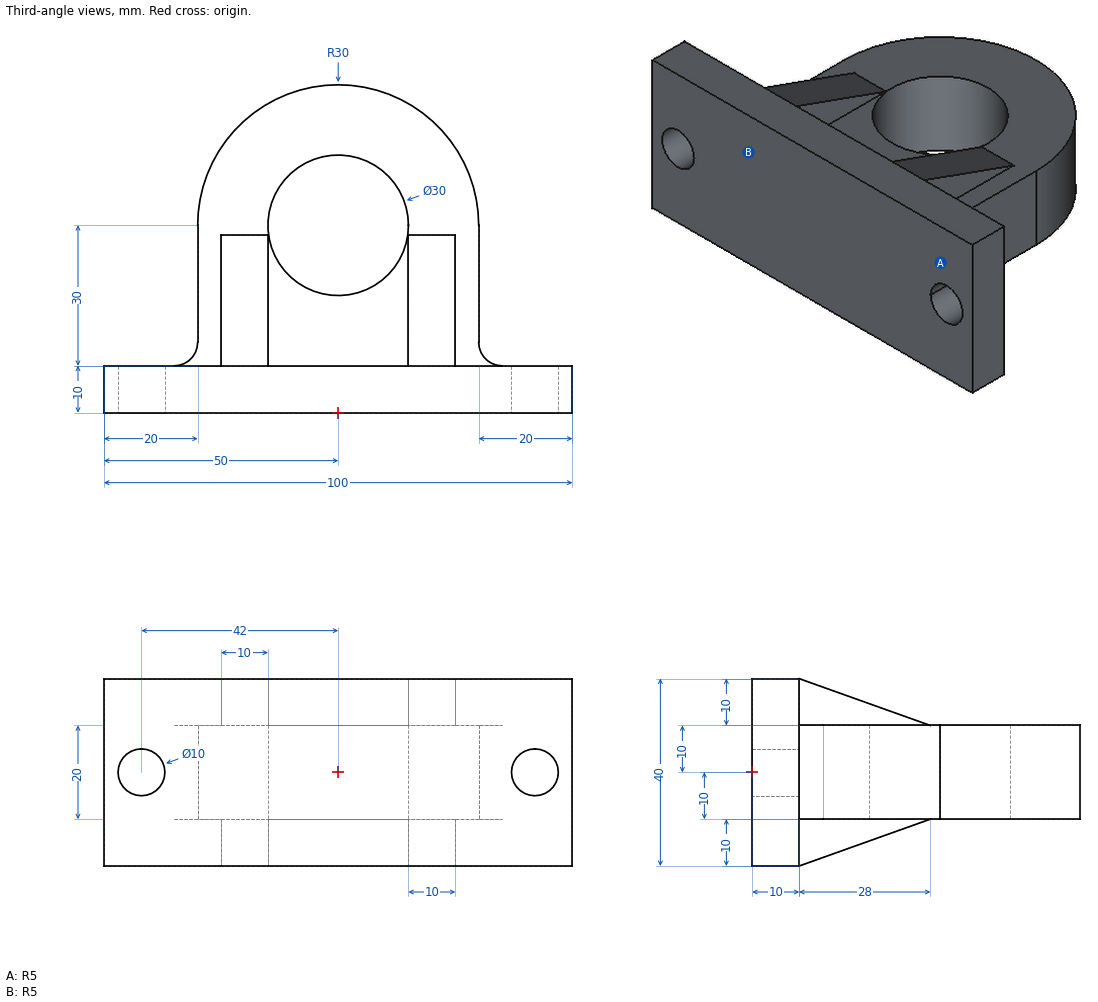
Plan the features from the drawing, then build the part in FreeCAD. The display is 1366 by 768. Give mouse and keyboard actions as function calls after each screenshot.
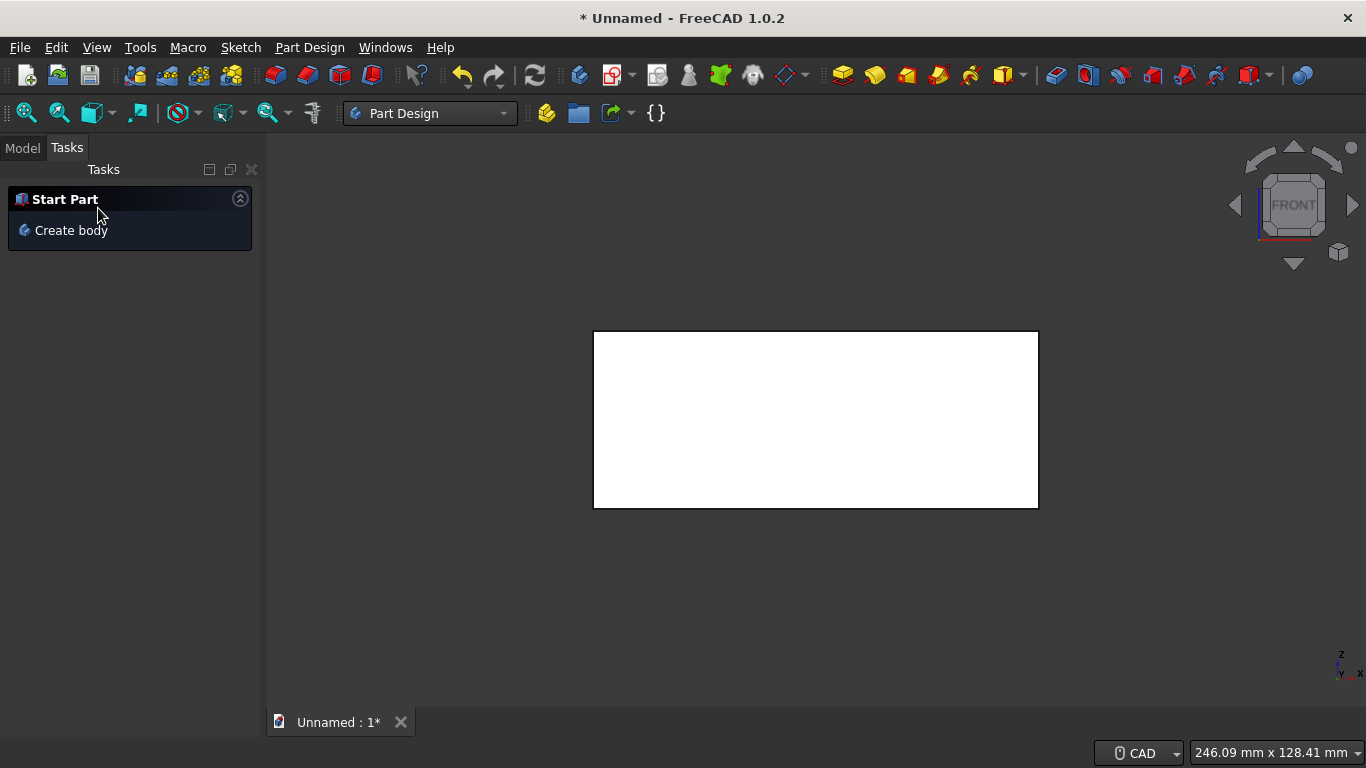
click(28, 114)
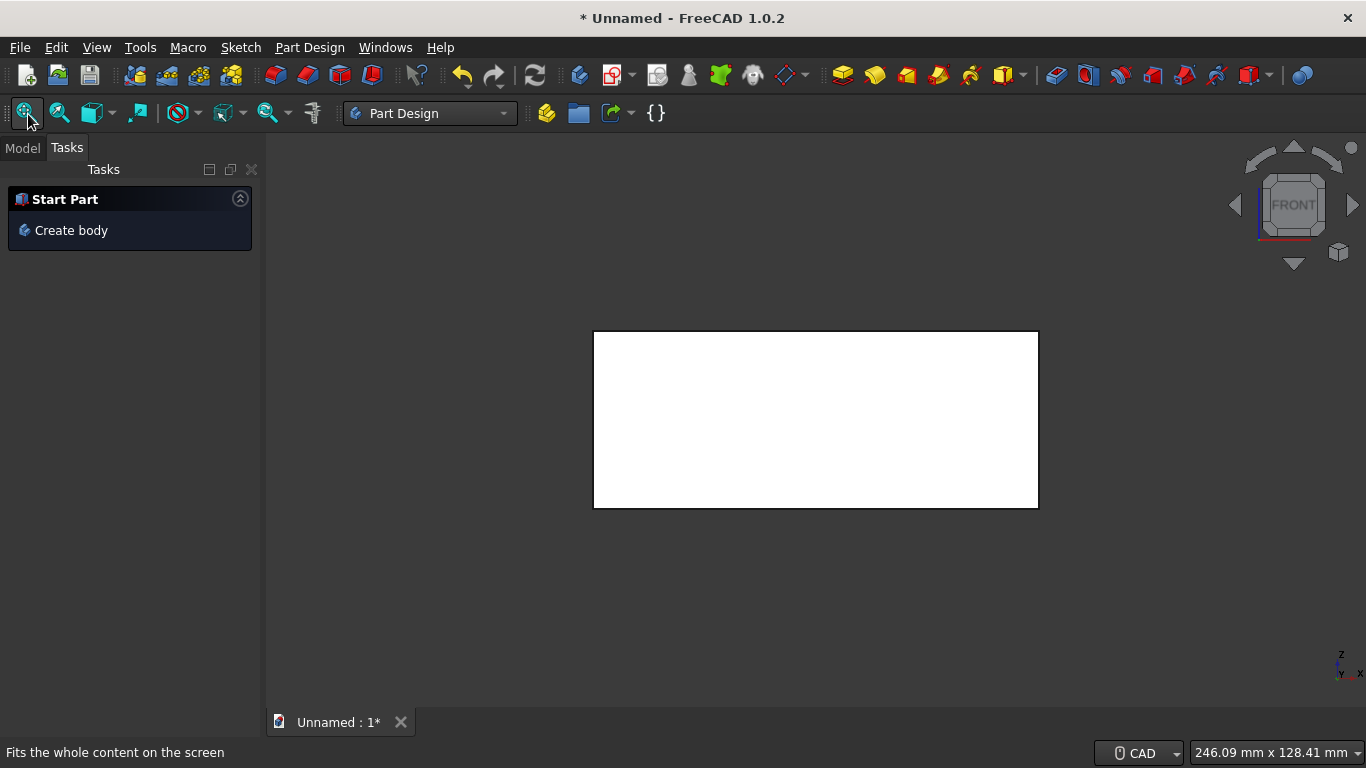
key(3)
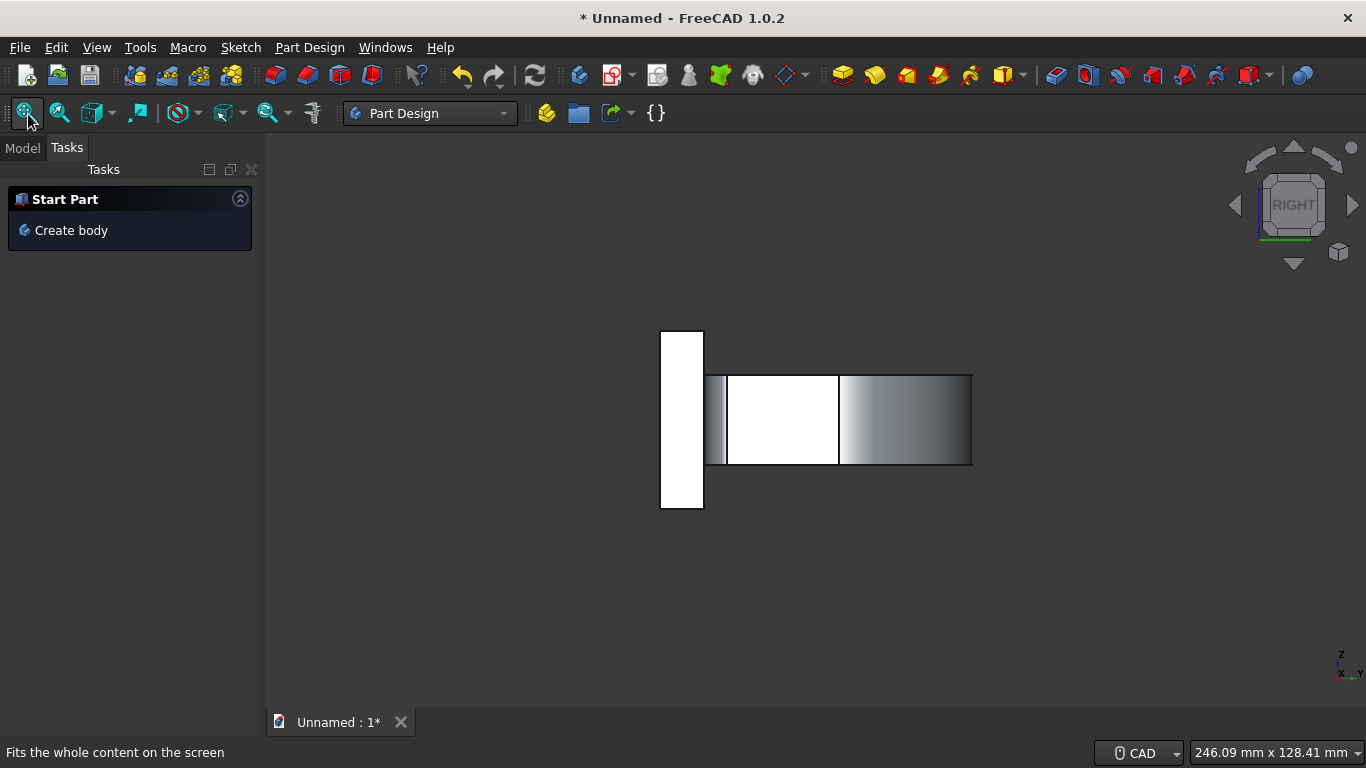
click(28, 114)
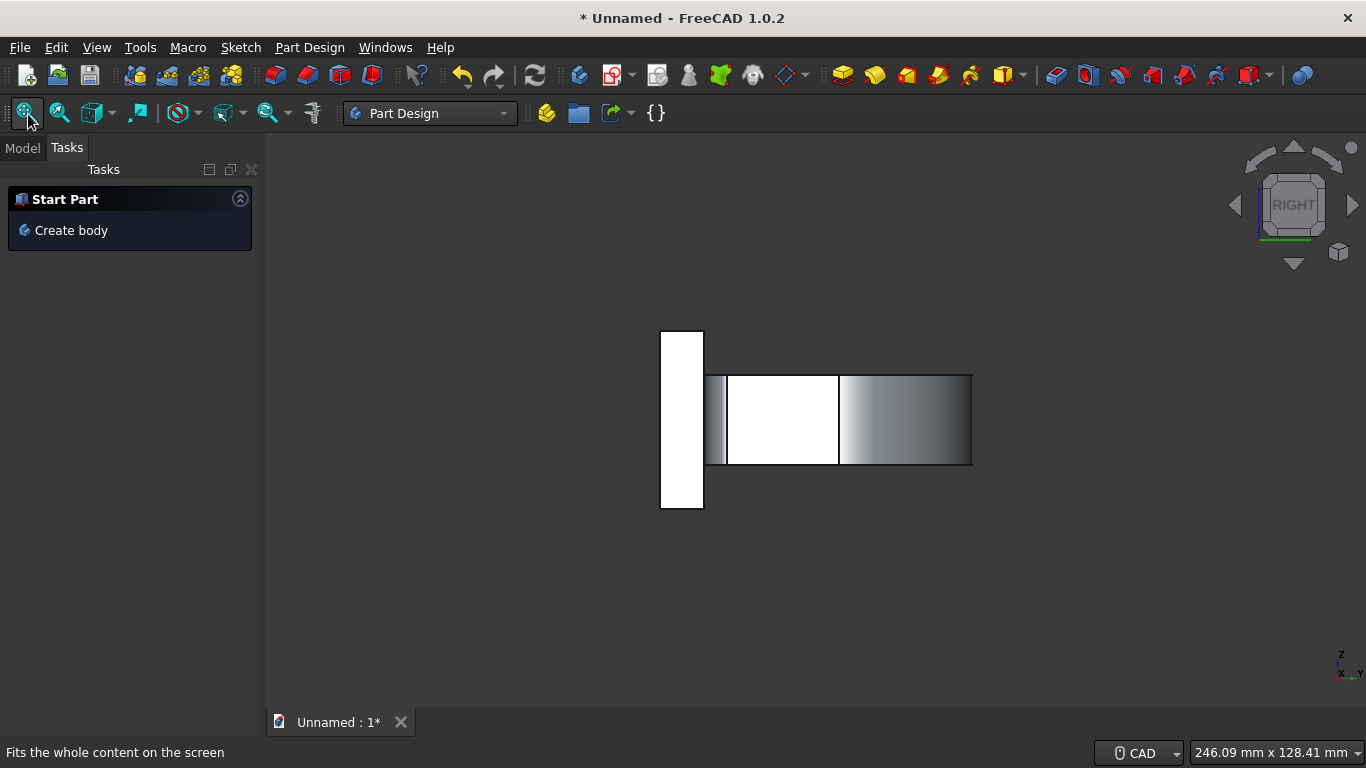
key(5)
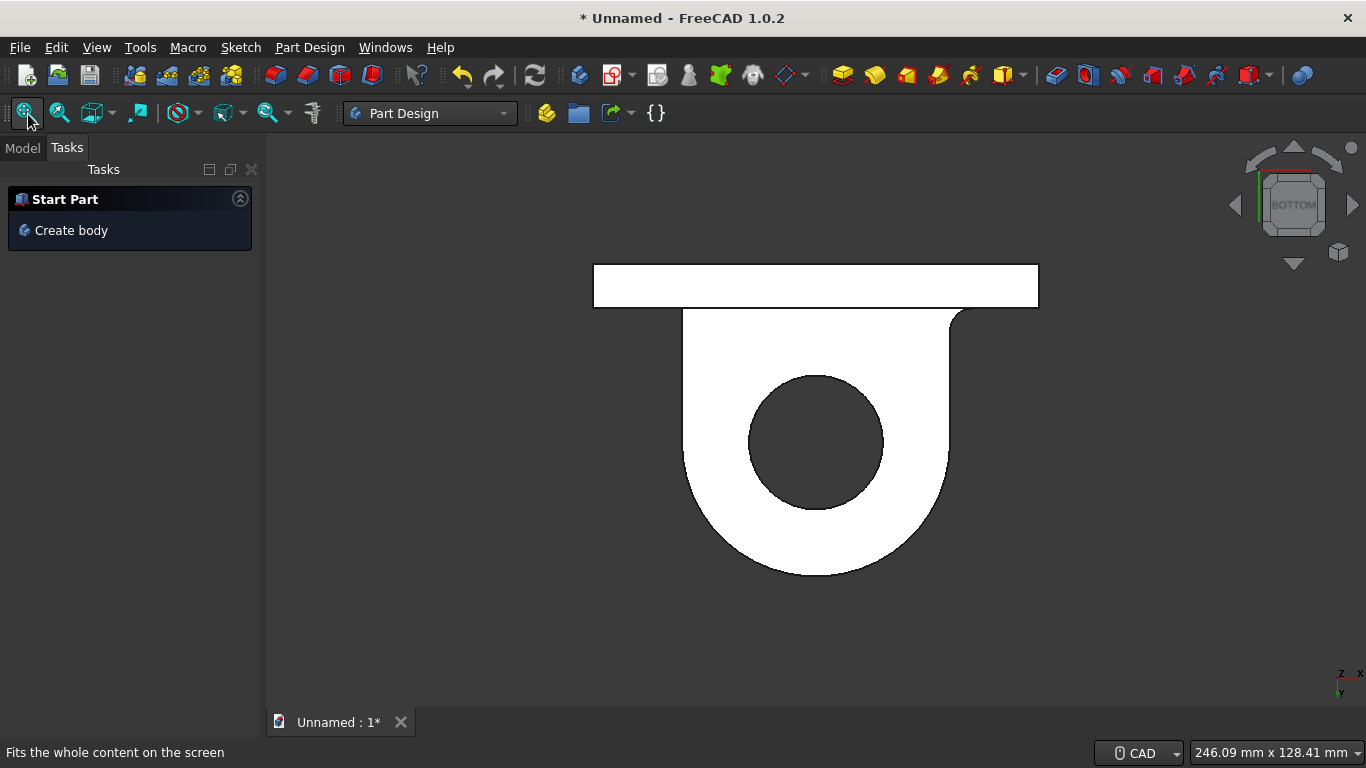
key(4)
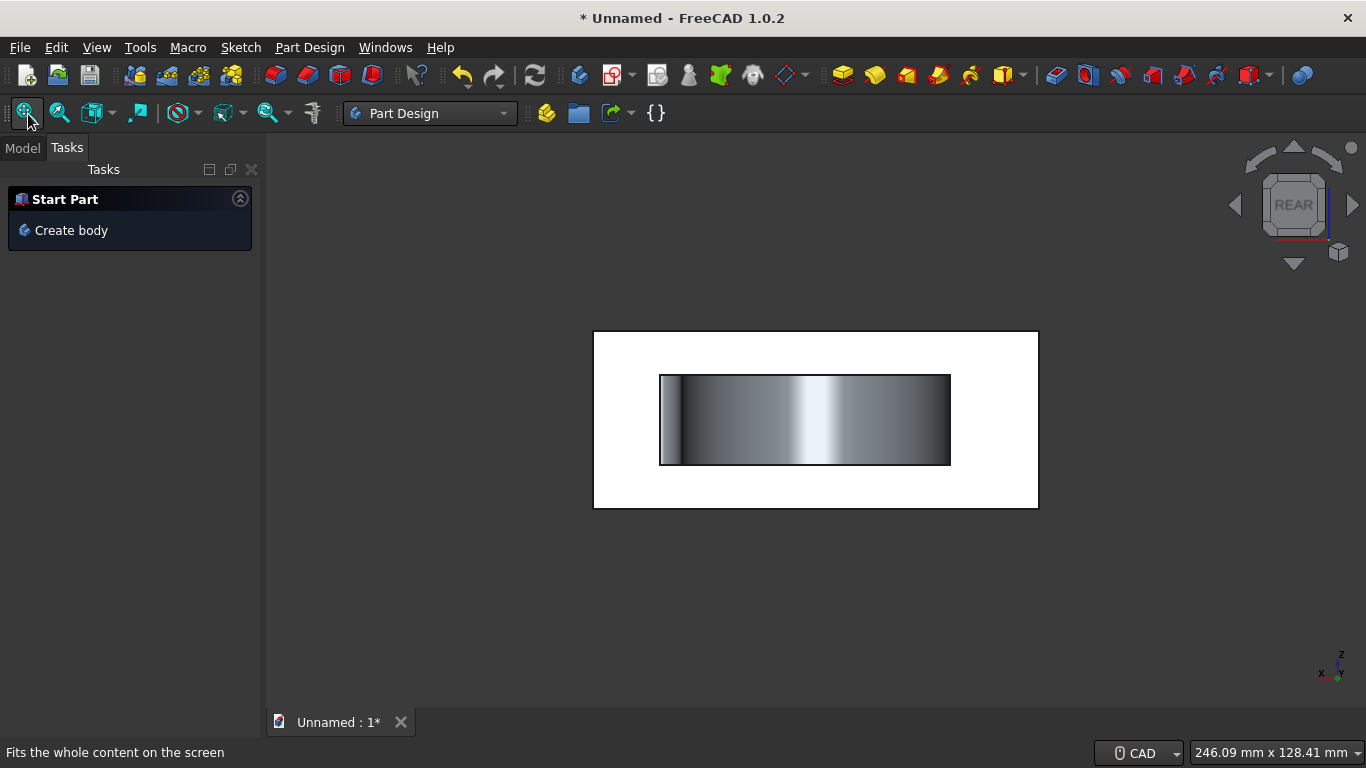
click(28, 114)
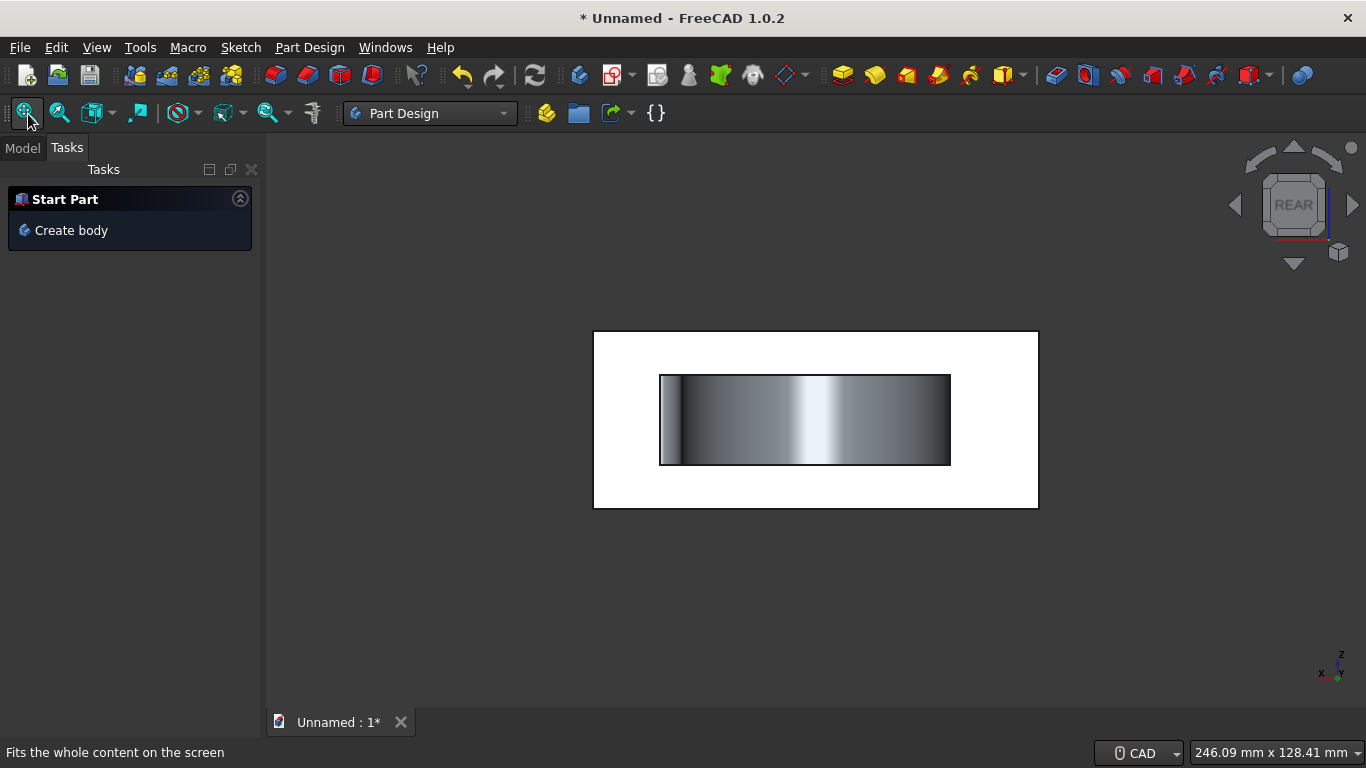
key(6)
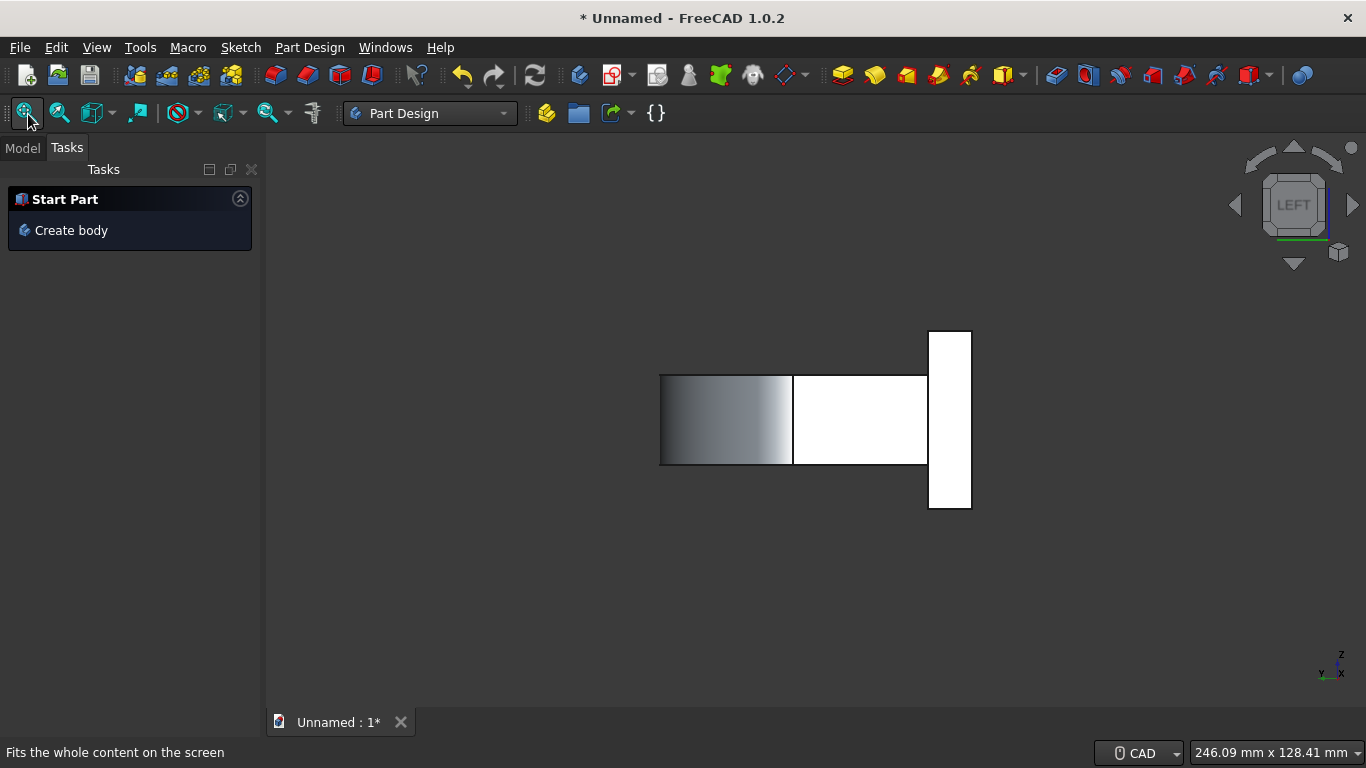
click(28, 114)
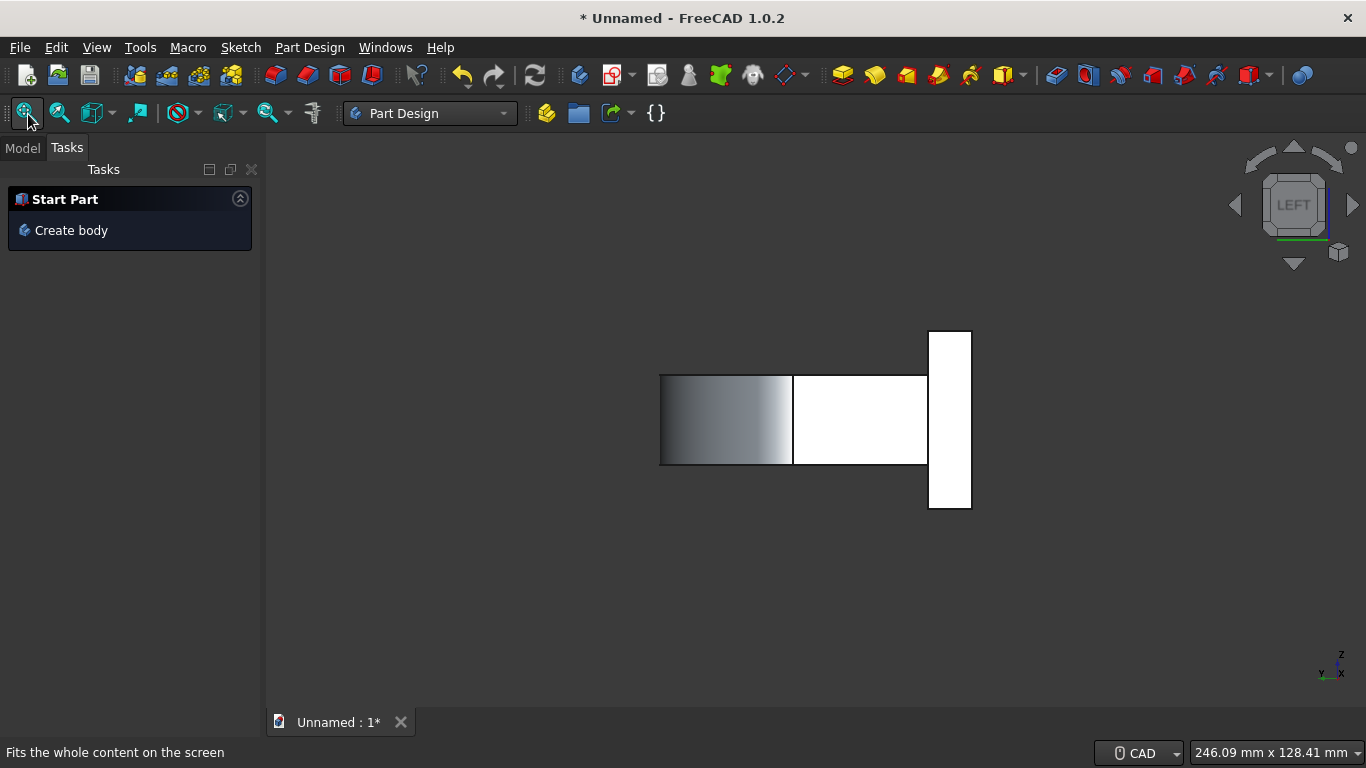
key(v)
key(3)